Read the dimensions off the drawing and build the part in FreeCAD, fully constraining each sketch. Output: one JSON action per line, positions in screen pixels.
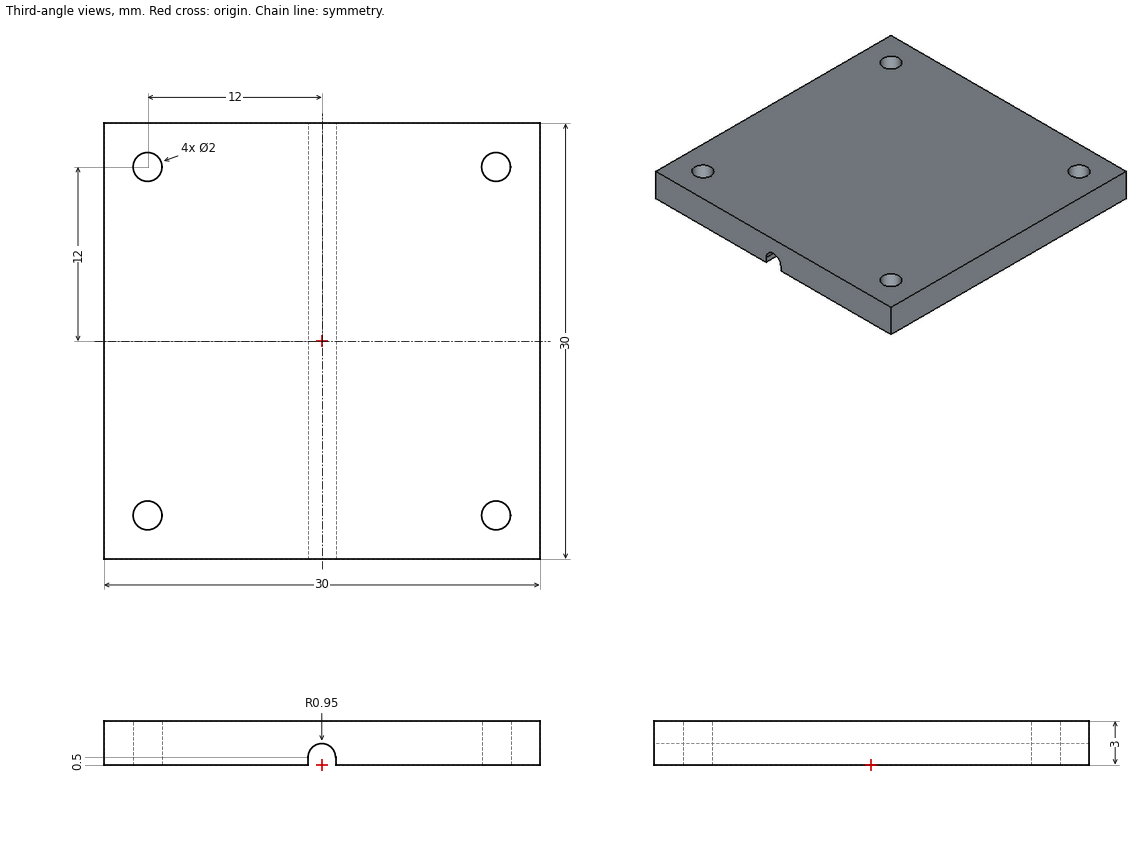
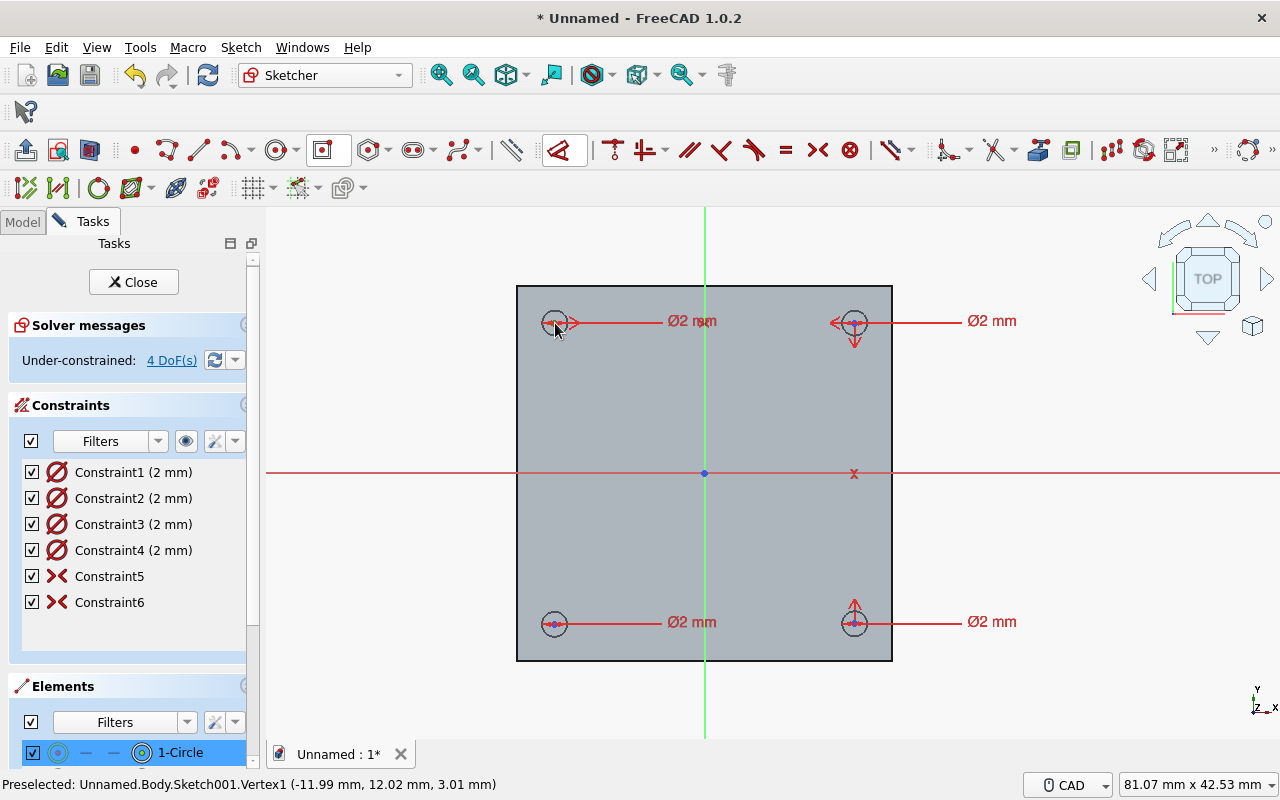
{"action": "left_click", "coordinate": [555, 624]}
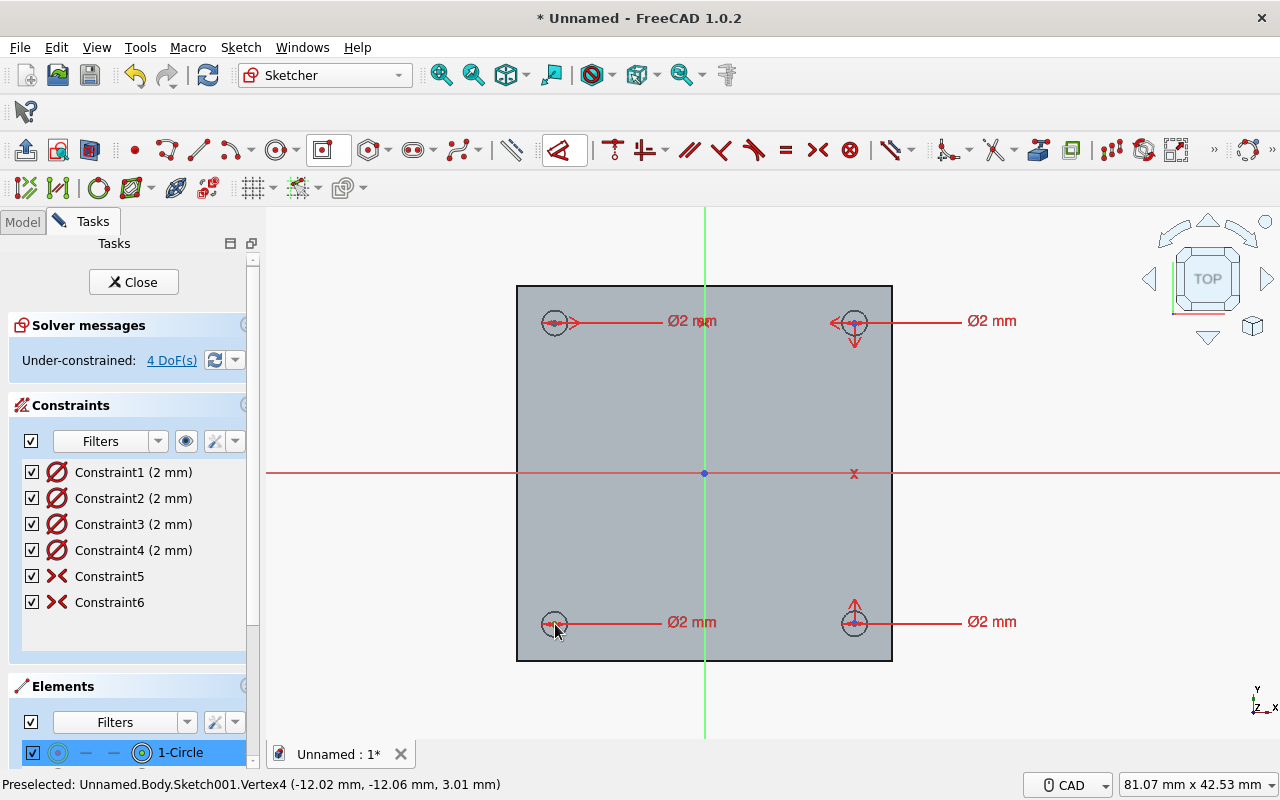
{"action": "left_click", "coordinate": [353, 473]}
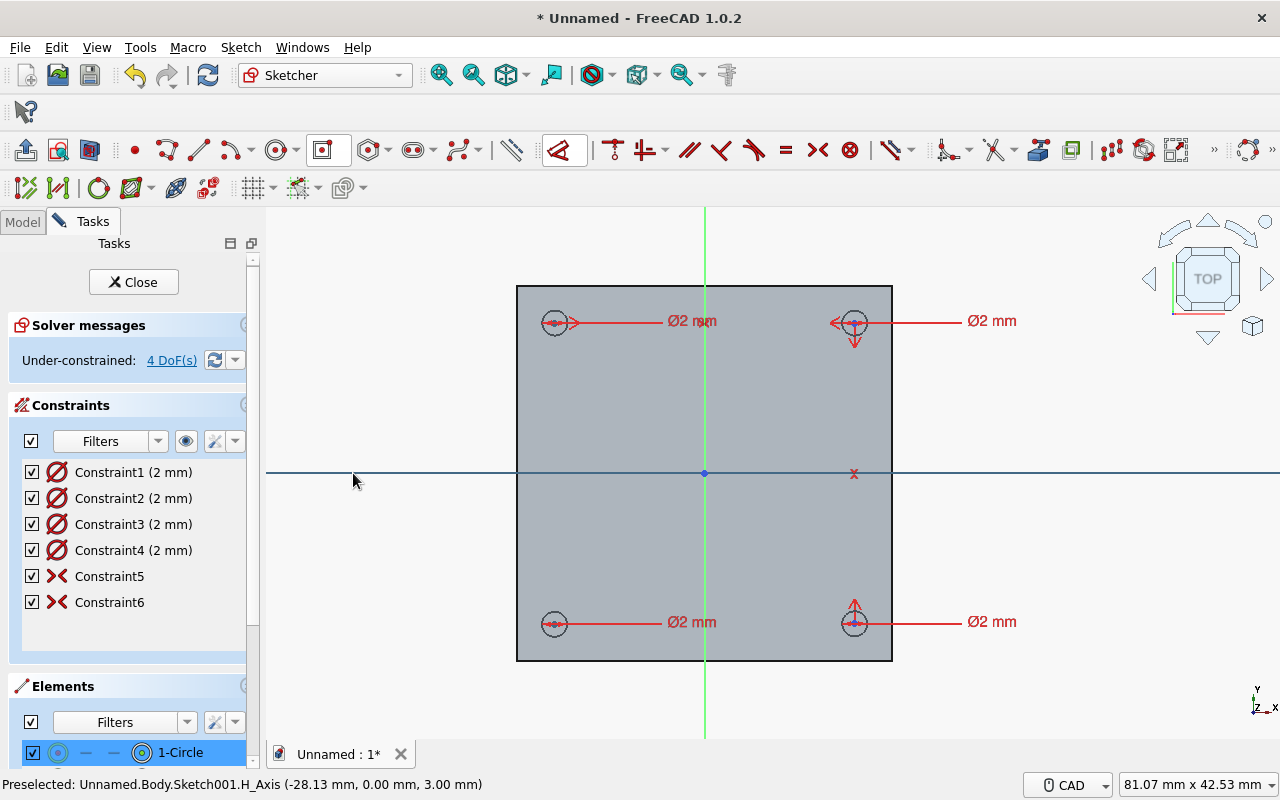
{"action": "key", "text": "s"}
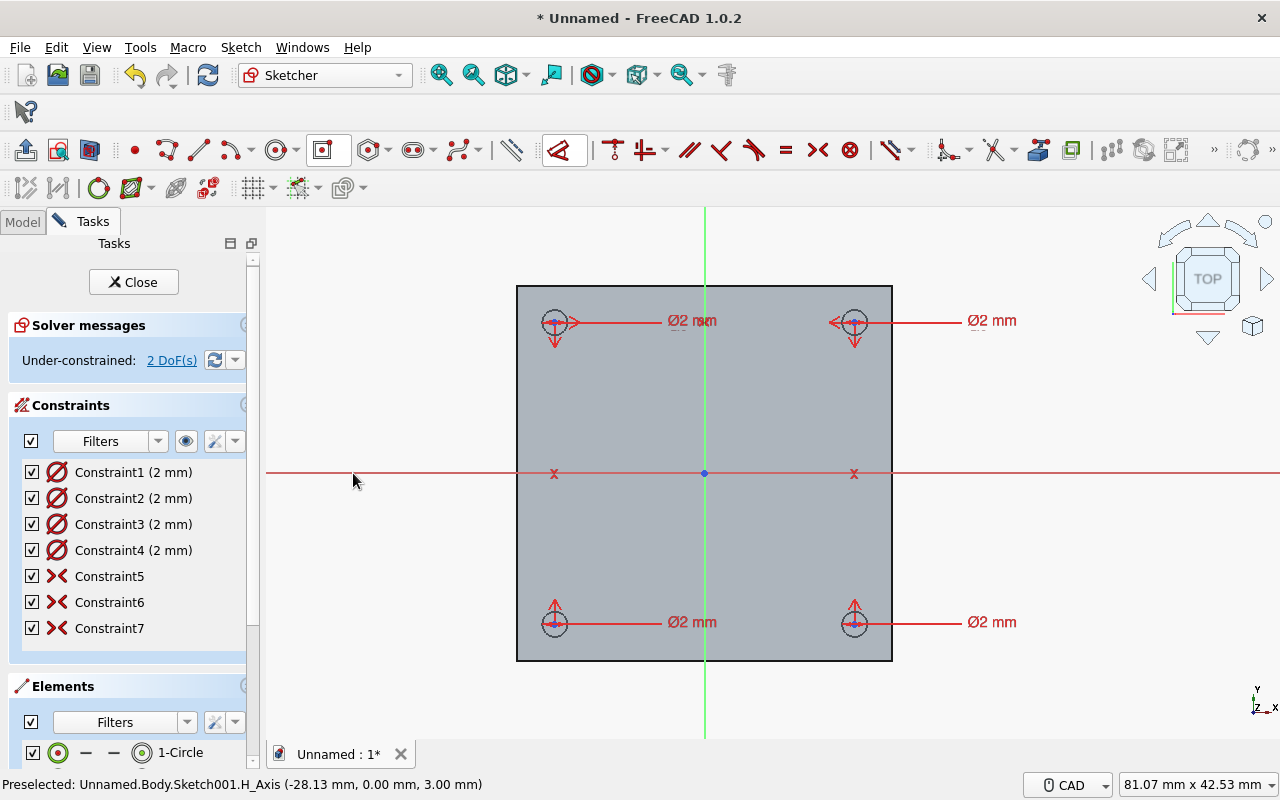
{"action": "left_click", "coordinate": [558, 150]}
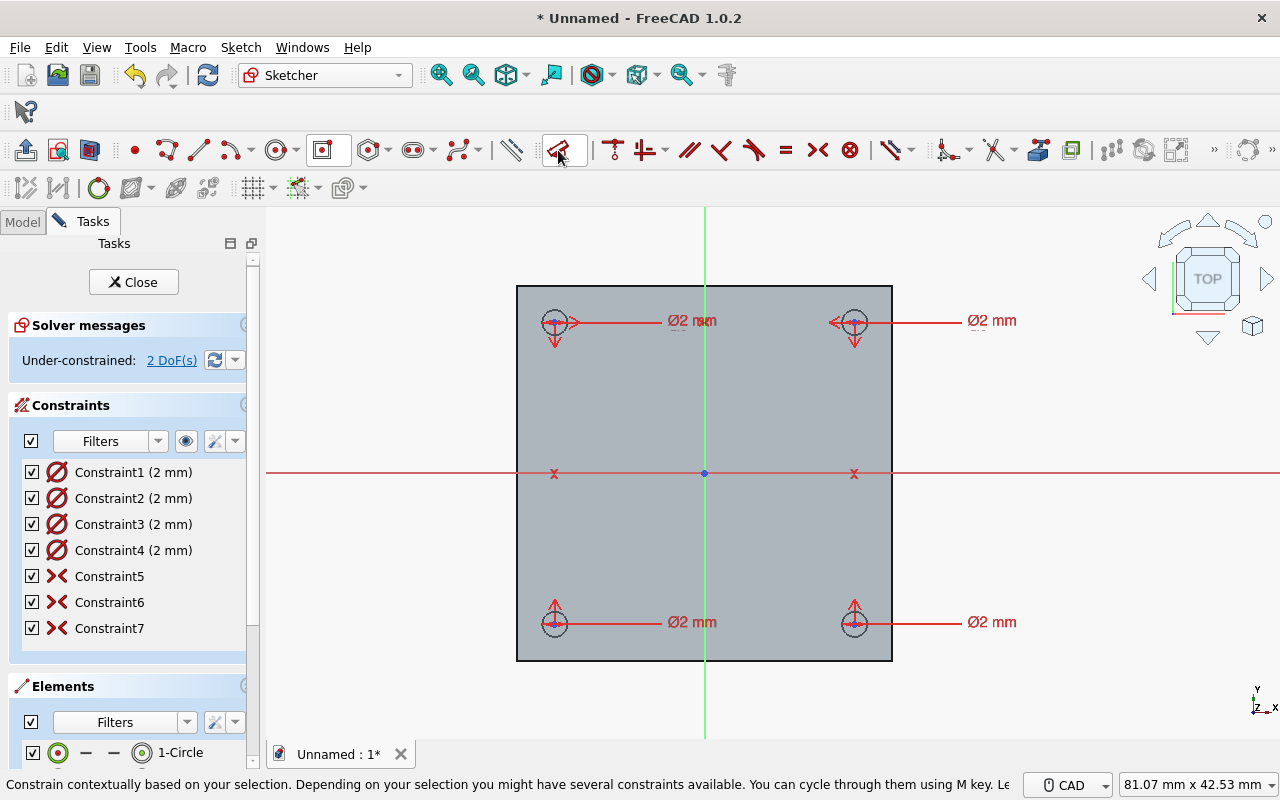
{"action": "left_click", "coordinate": [555, 323]}
{"action": "left_click", "coordinate": [630, 289]}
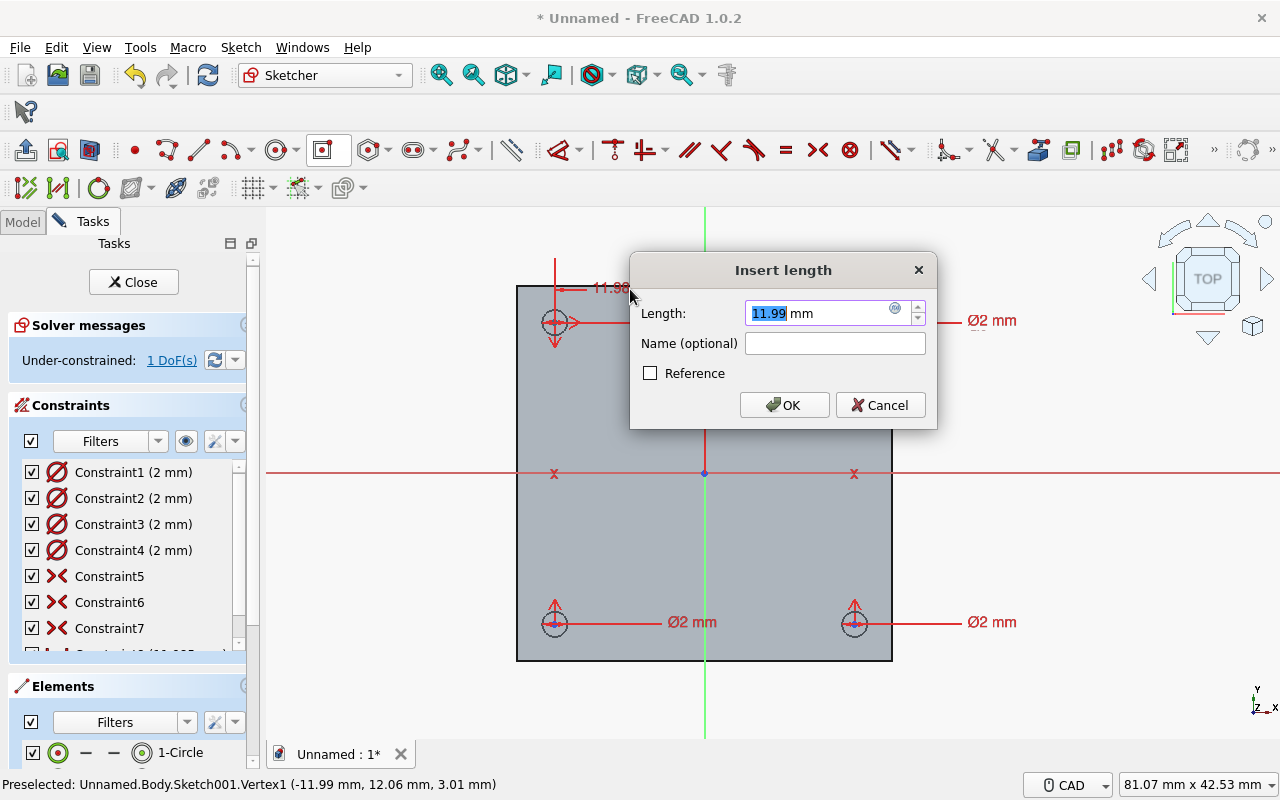
{"action": "type", "text": "12"}
{"action": "key", "text": "Return"}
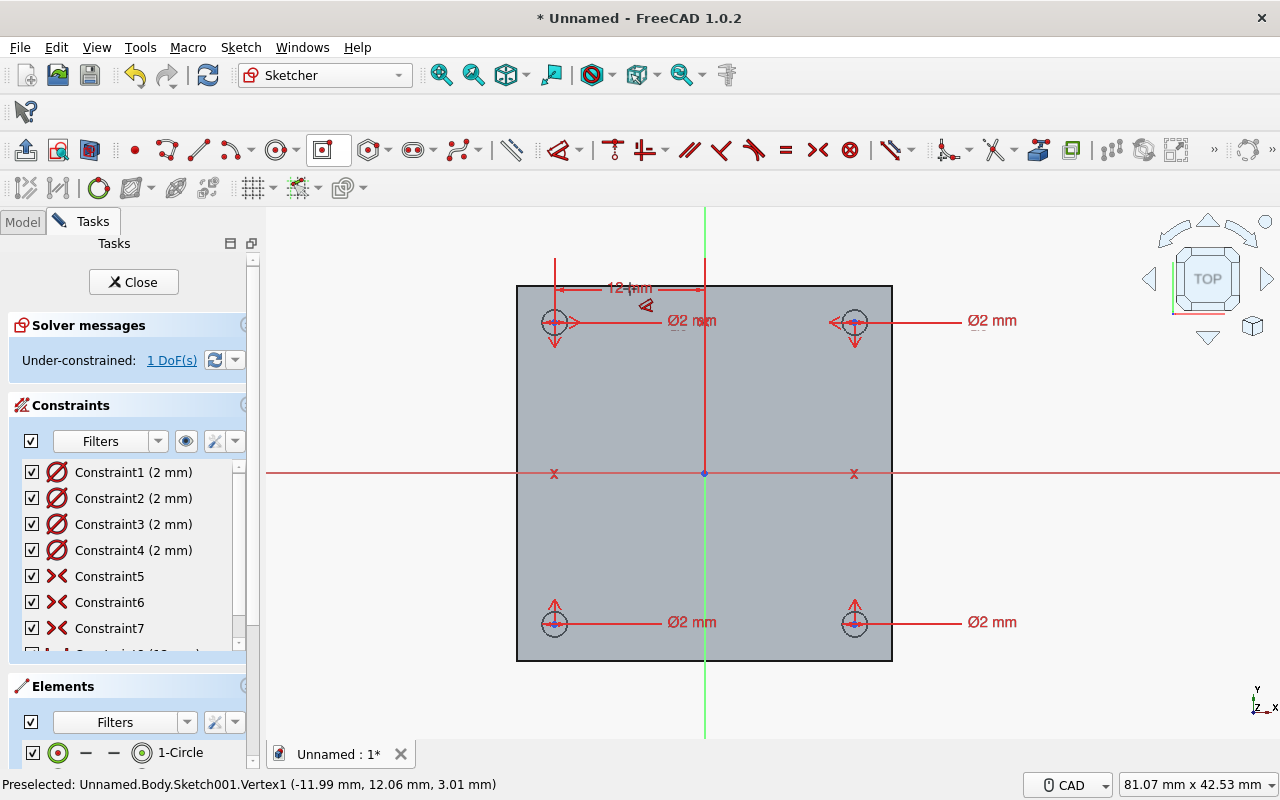
{"action": "left_click", "coordinate": [555, 323]}
{"action": "left_click", "coordinate": [521, 398]}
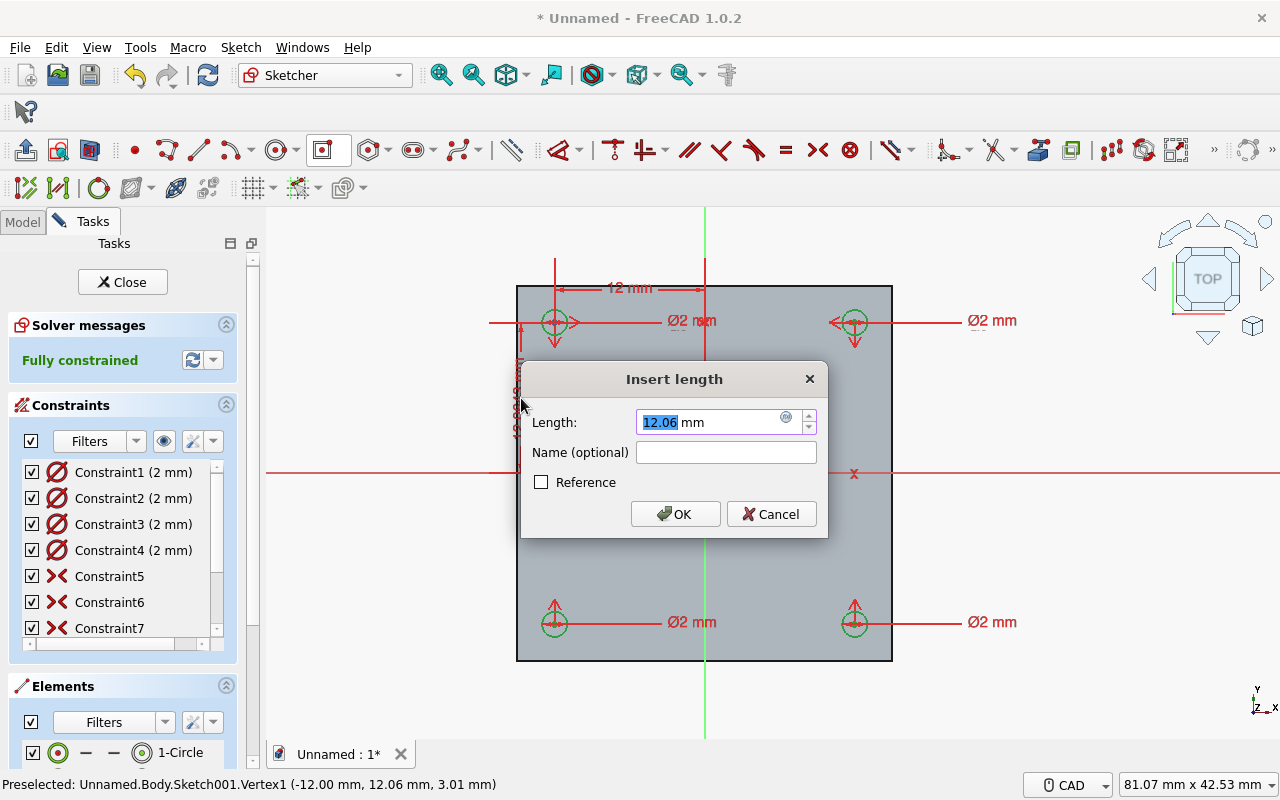
{"action": "type", "text": "12"}
{"action": "key", "text": "Return"}
{"action": "key", "text": "Escape"}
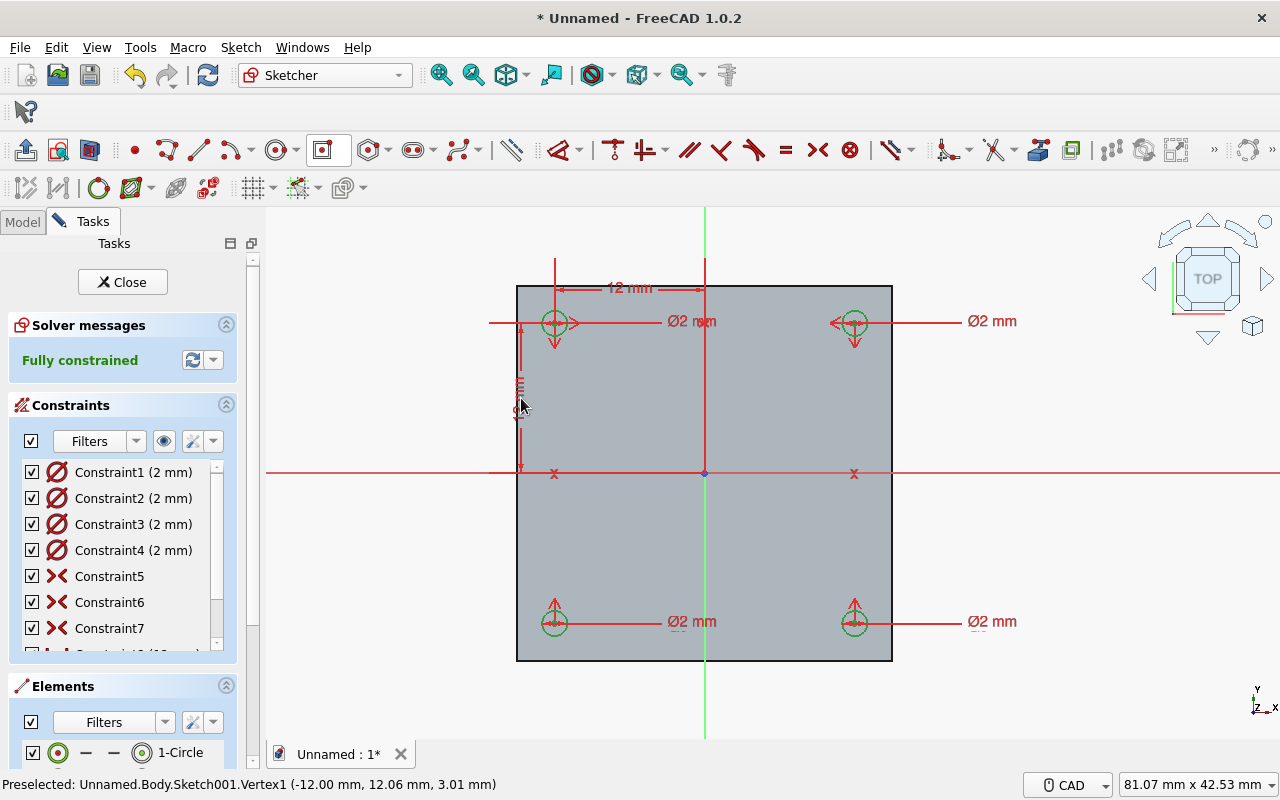
{"action": "left_click", "coordinate": [123, 282]}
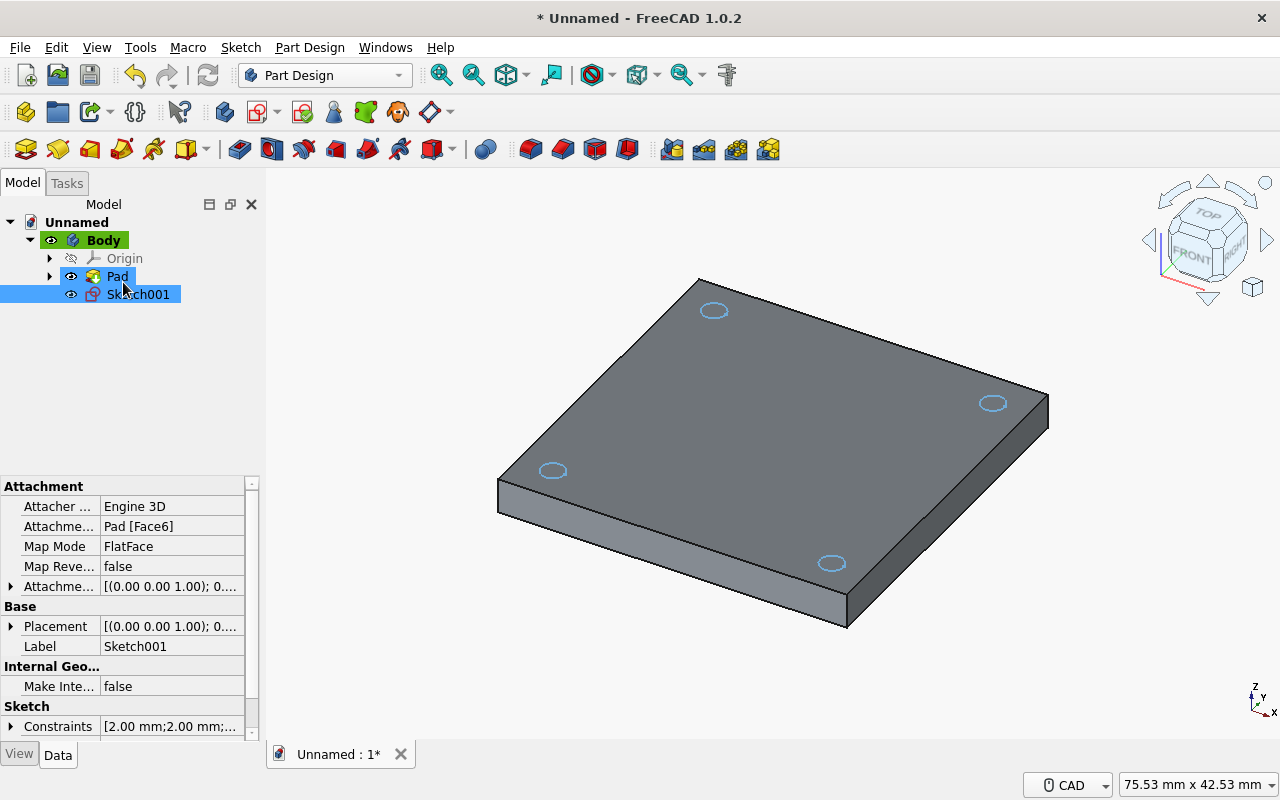
{"action": "left_click", "coordinate": [240, 150]}